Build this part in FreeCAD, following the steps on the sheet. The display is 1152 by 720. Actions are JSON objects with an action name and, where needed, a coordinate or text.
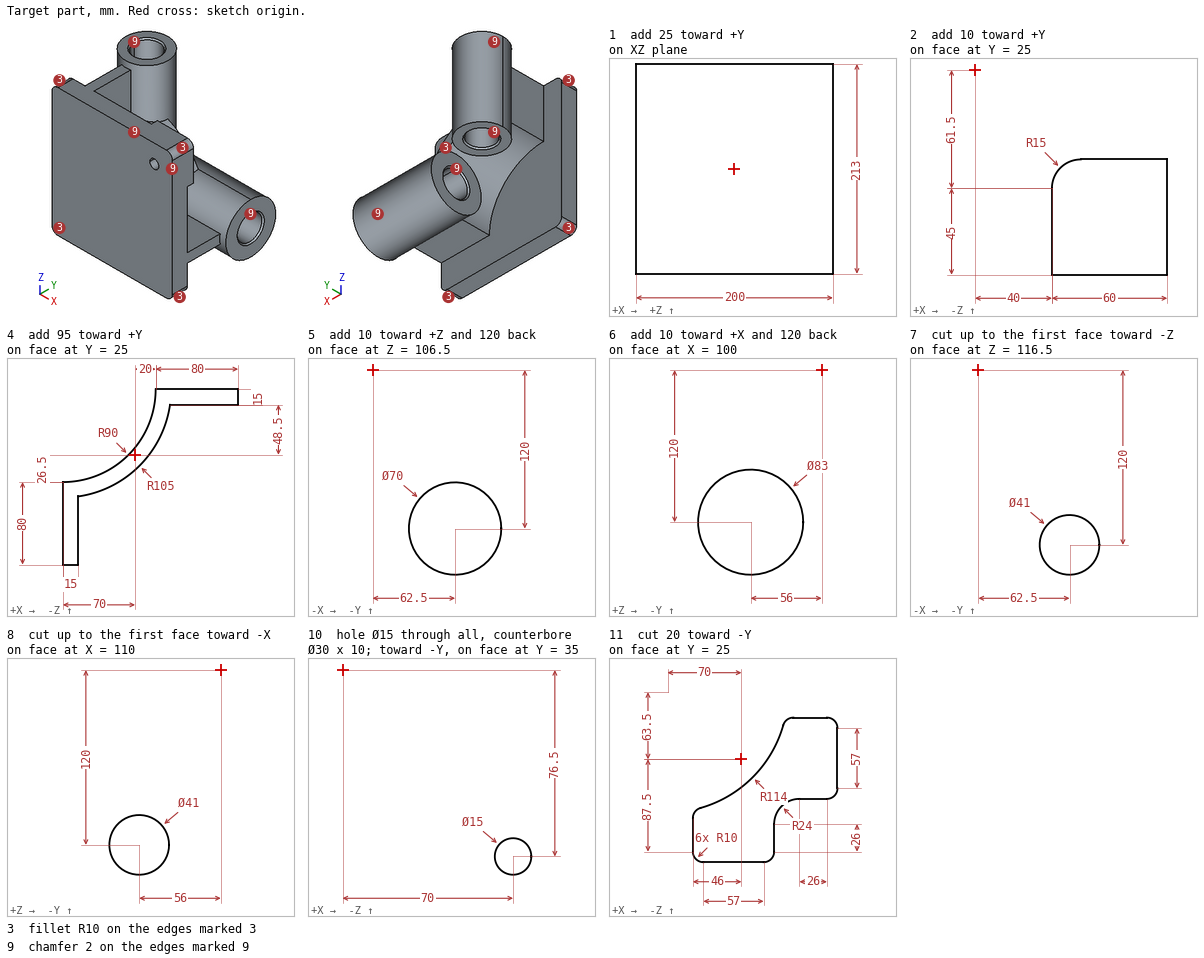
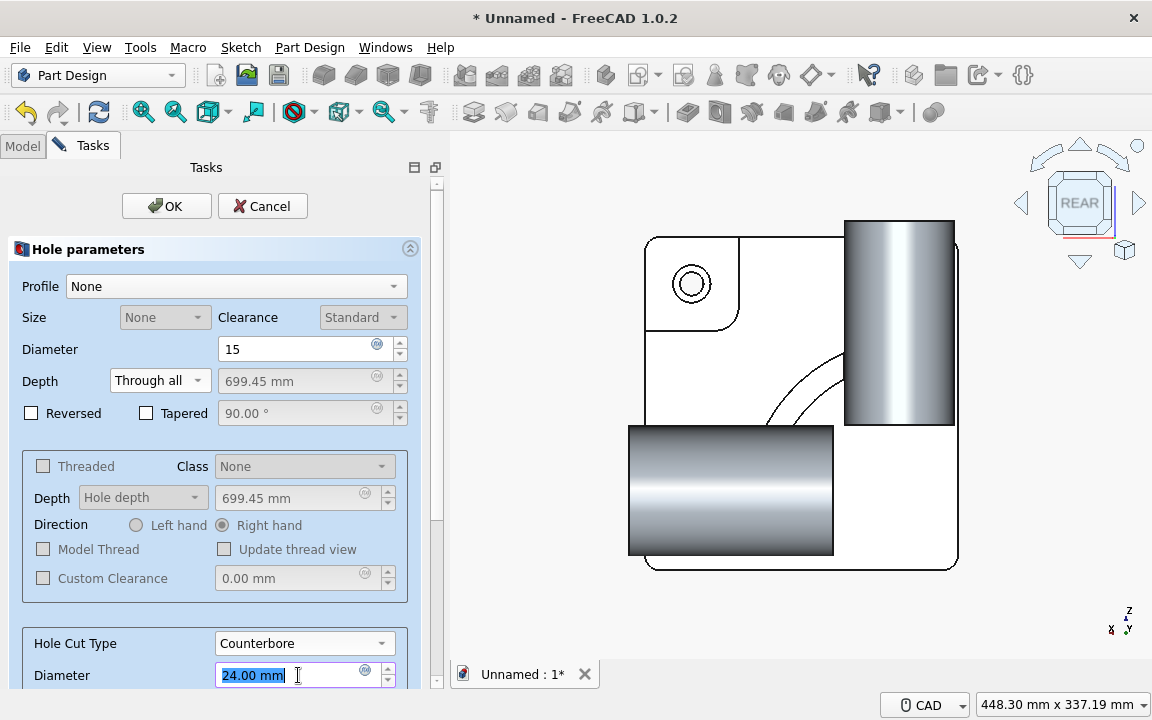
{"action": "type", "text": "30"}
{"action": "key", "text": "Tab"}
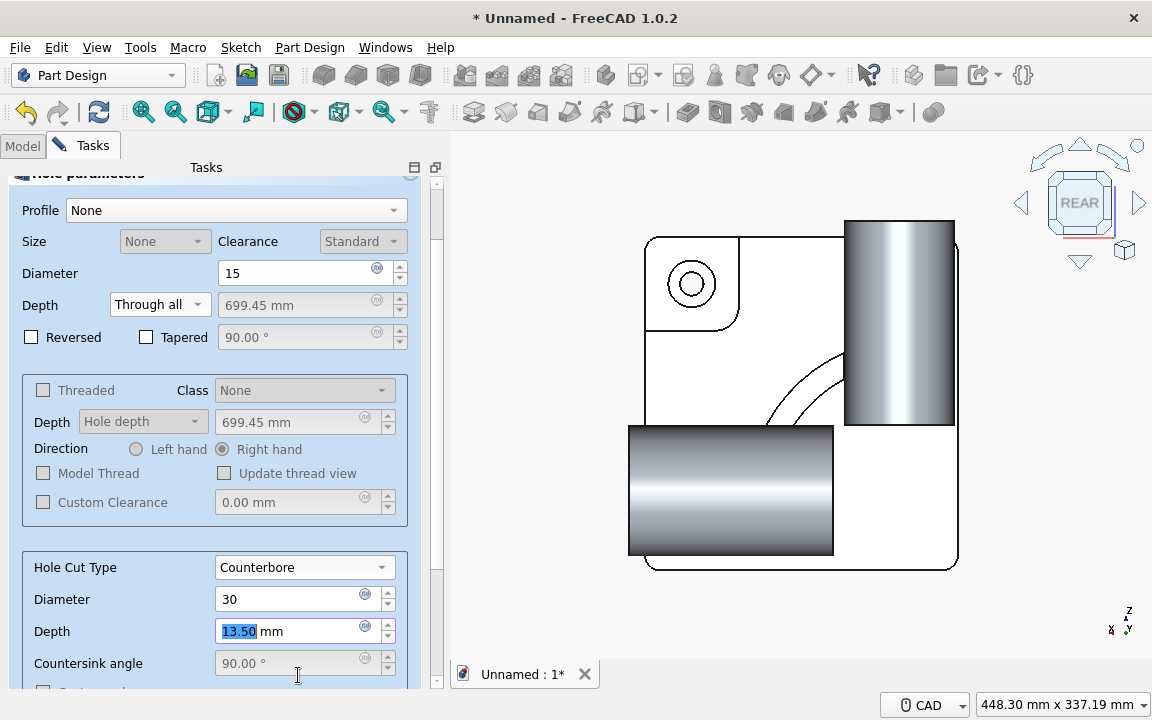
{"action": "type", "text": "10"}
{"action": "key", "text": "Tab"}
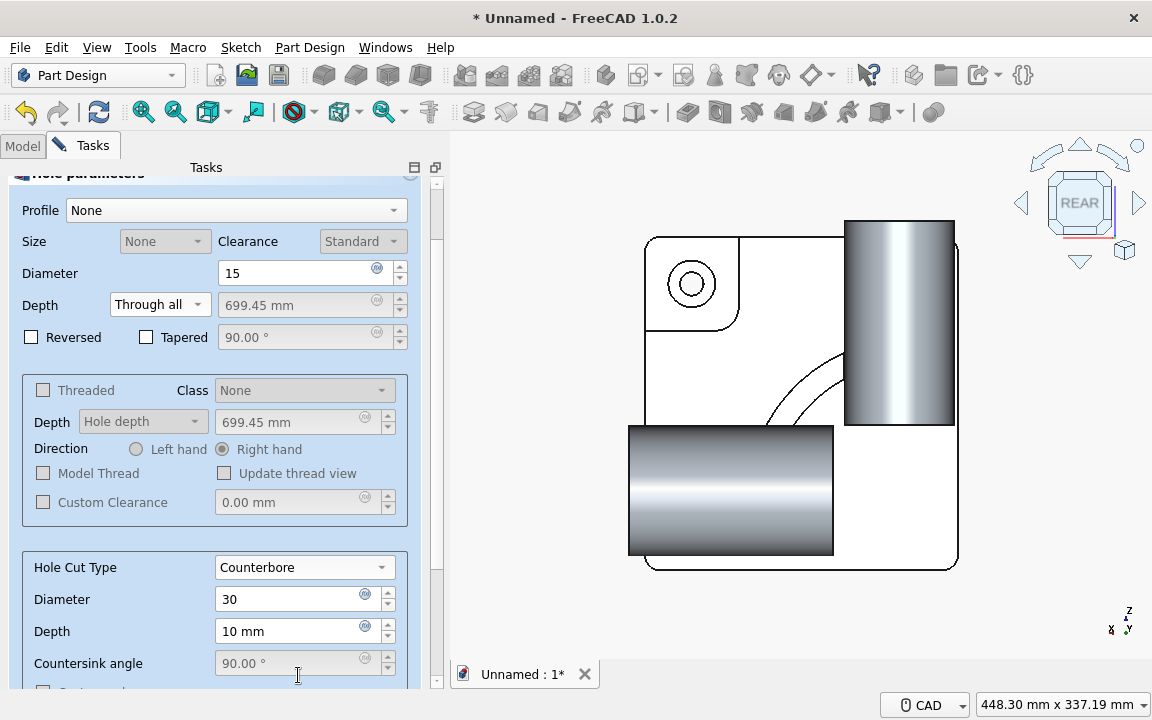
{"action": "scroll", "coordinate": [437, 432], "scroll_direction": "up", "scroll_amount": 3}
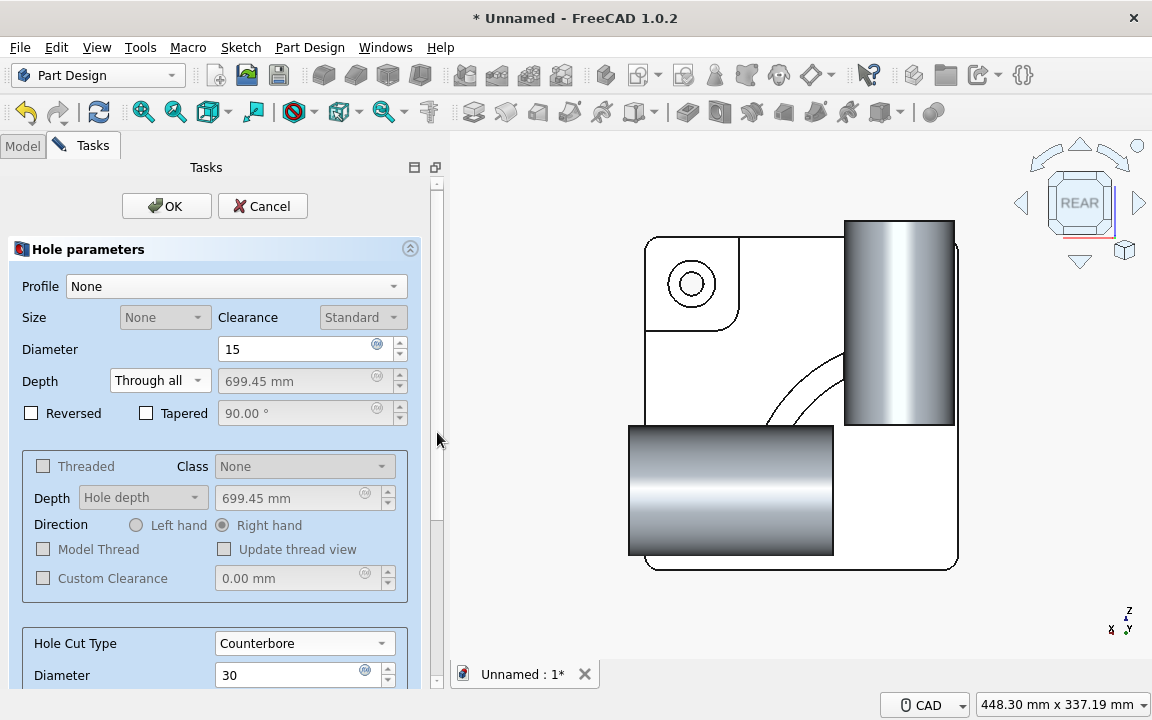
{"action": "left_click", "coordinate": [167, 206]}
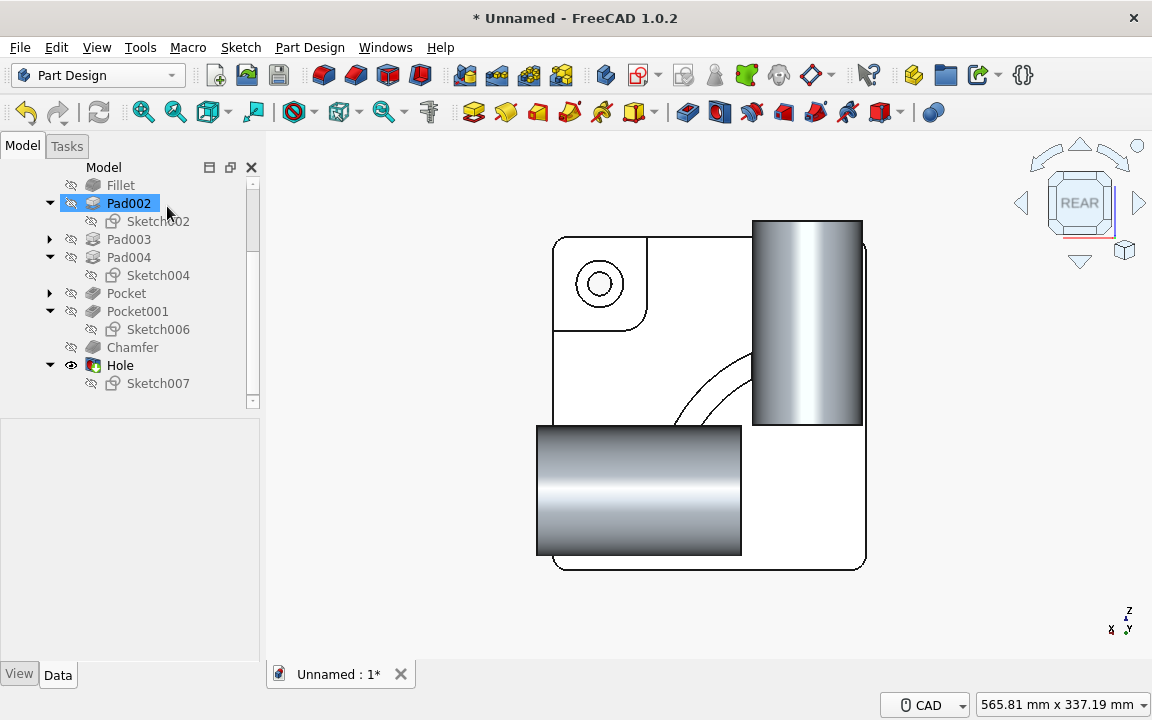
{"action": "left_click", "coordinate": [754, 498]}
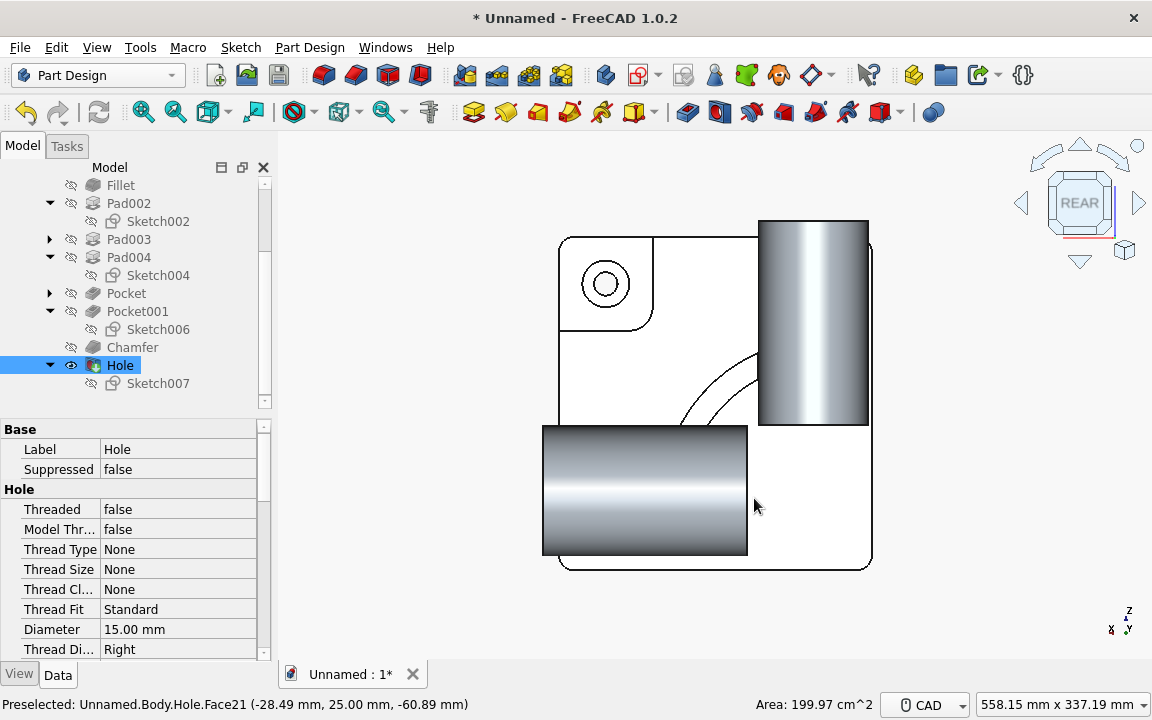
{"action": "left_click", "coordinate": [638, 76]}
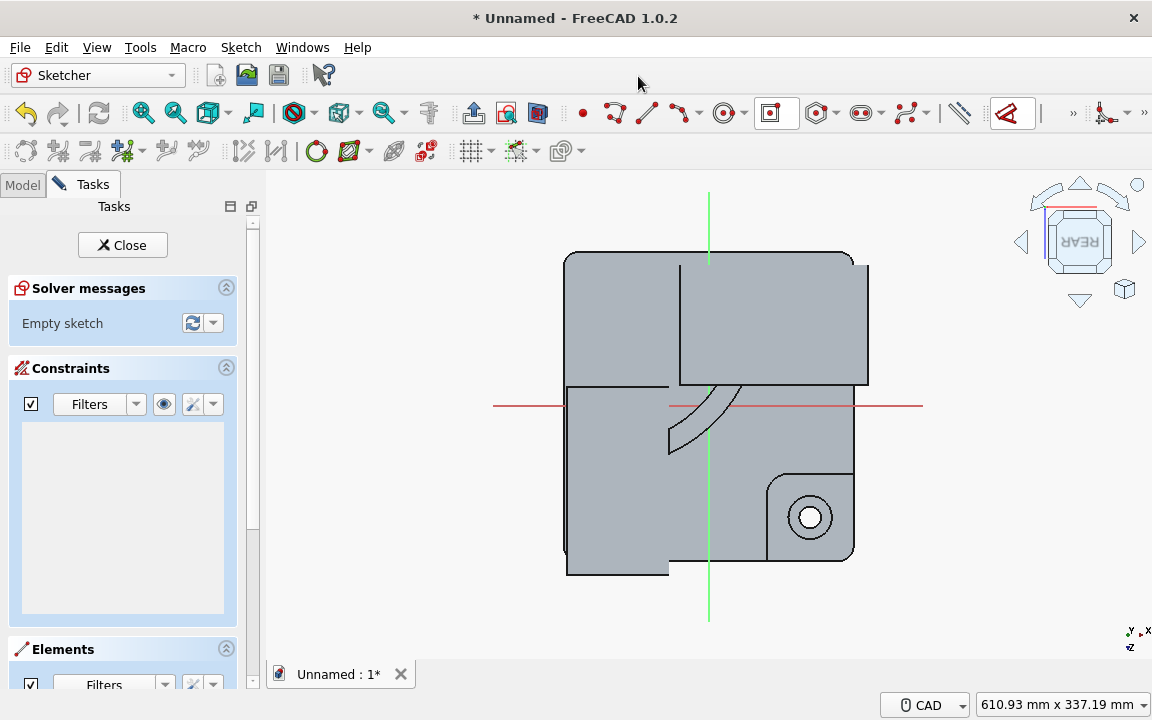
{"action": "left_click", "coordinate": [538, 114]}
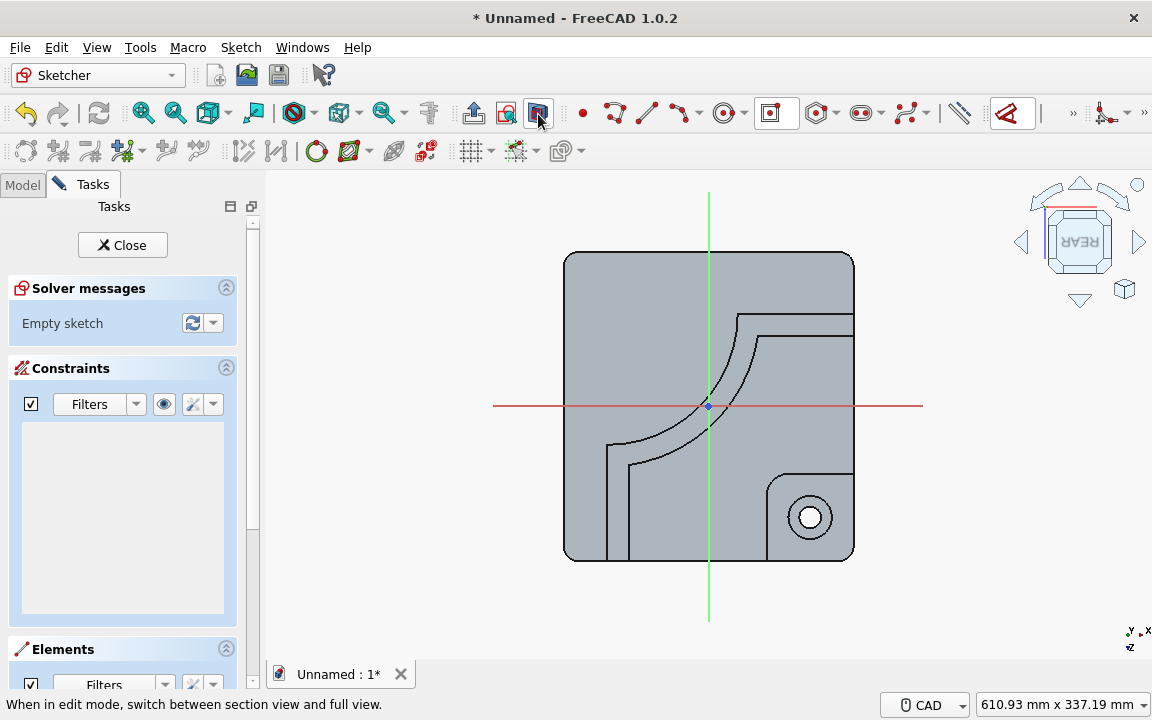
{"action": "scroll", "coordinate": [946, 518], "scroll_direction": "up", "scroll_amount": 2}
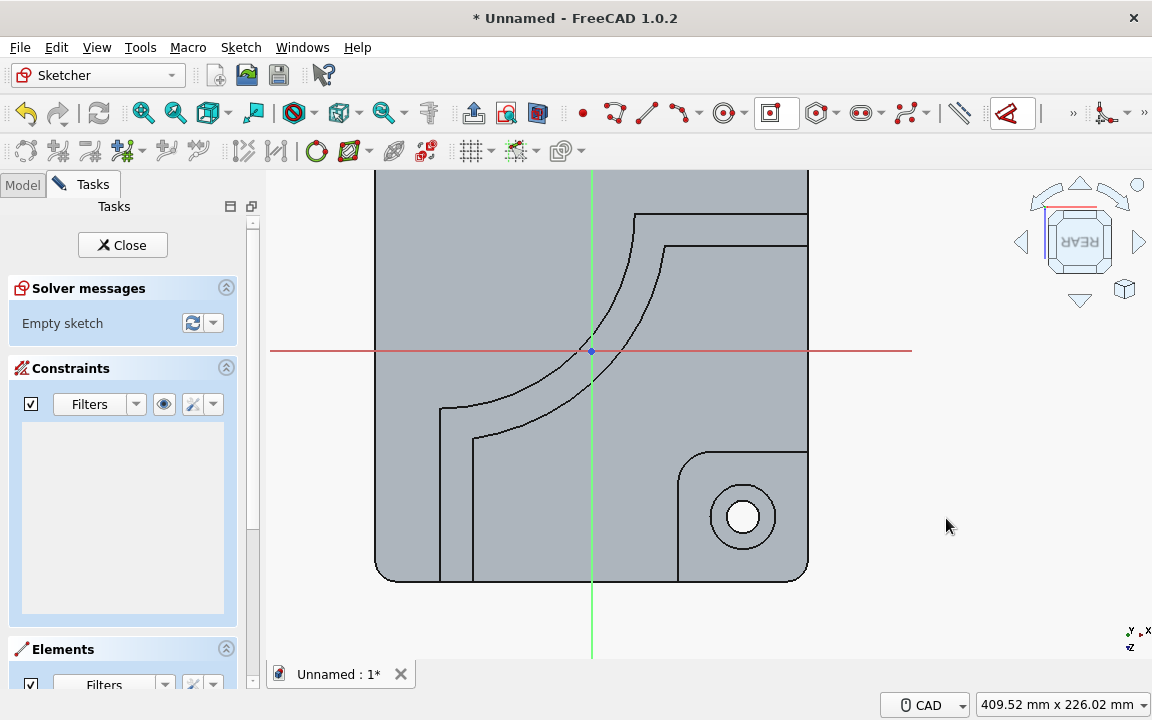
{"action": "left_click", "coordinate": [648, 114]}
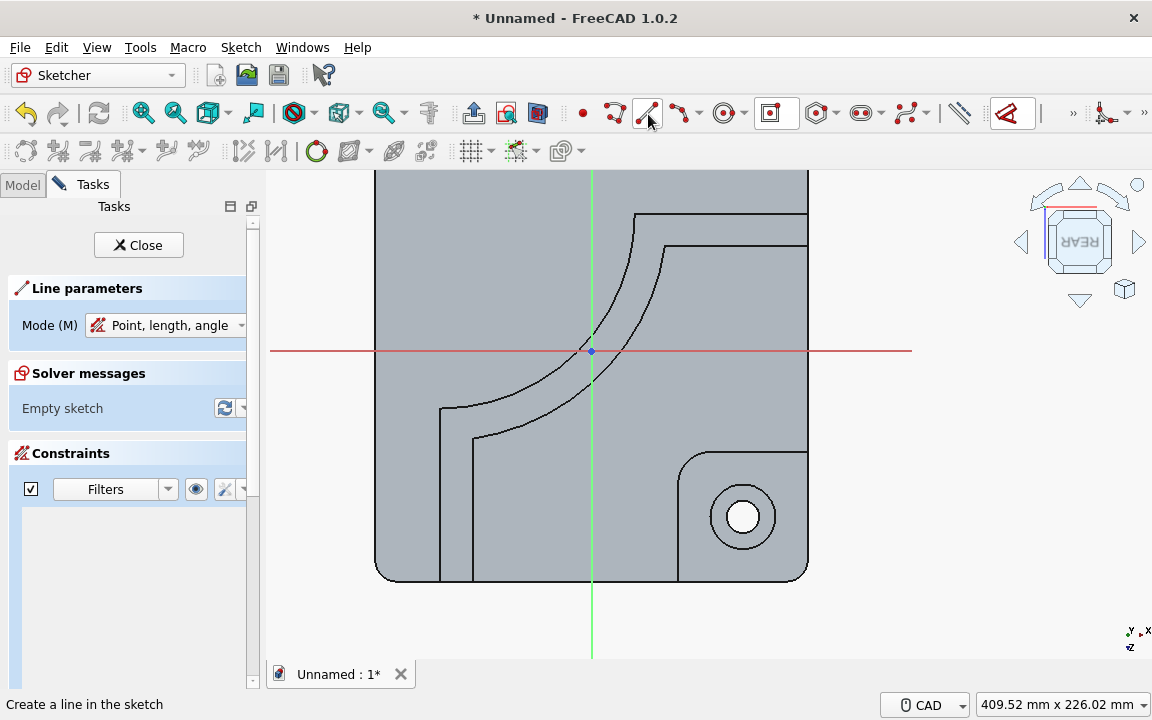
{"action": "left_click", "coordinate": [492, 472]}
{"action": "left_click", "coordinate": [492, 541]}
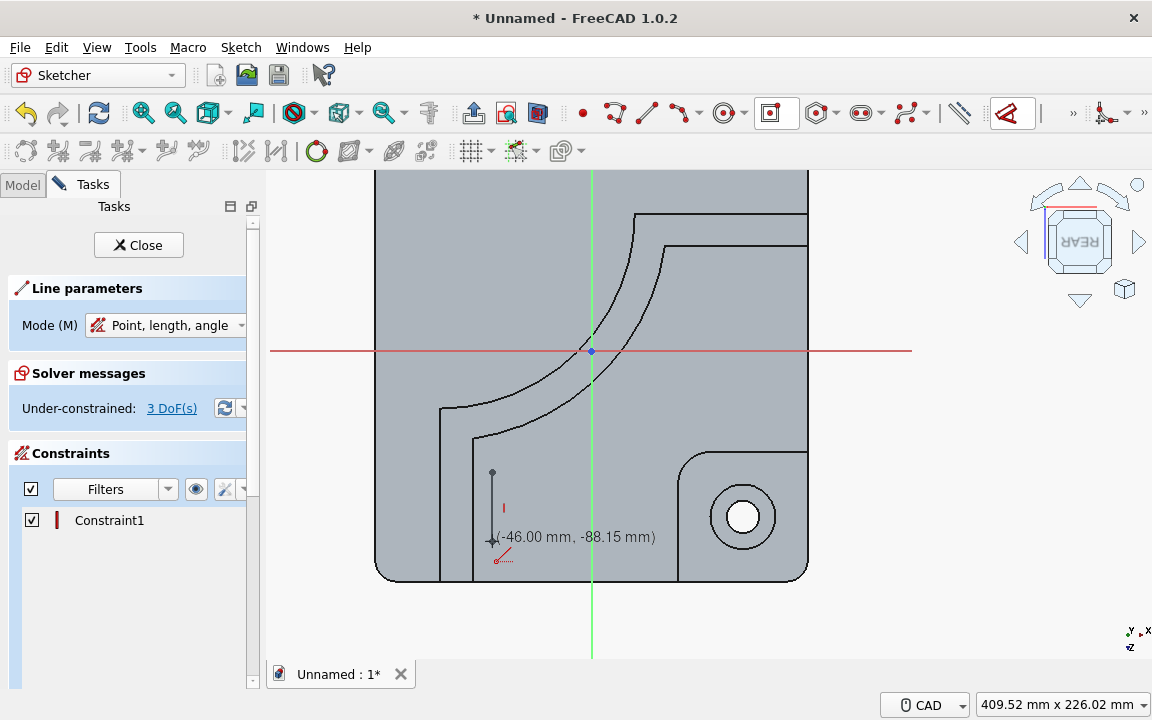
{"action": "left_click", "coordinate": [514, 562]}
{"action": "left_click", "coordinate": [637, 562]}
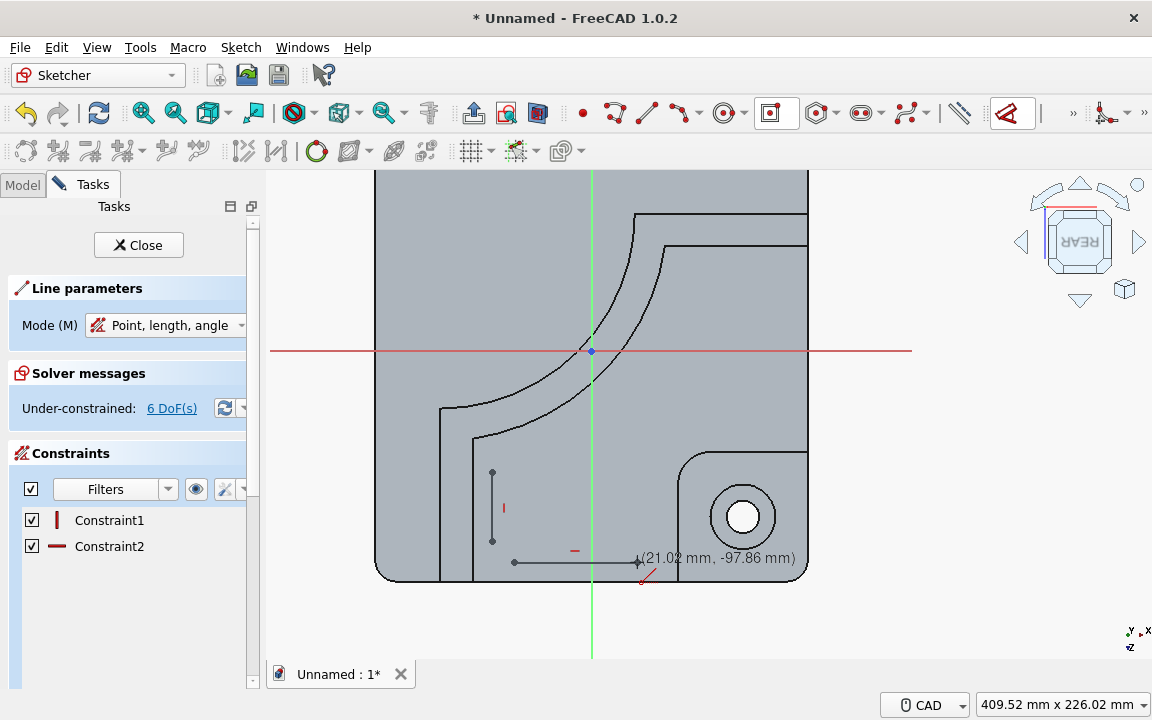
{"action": "left_click", "coordinate": [659, 541]}
{"action": "left_click", "coordinate": [659, 484]}